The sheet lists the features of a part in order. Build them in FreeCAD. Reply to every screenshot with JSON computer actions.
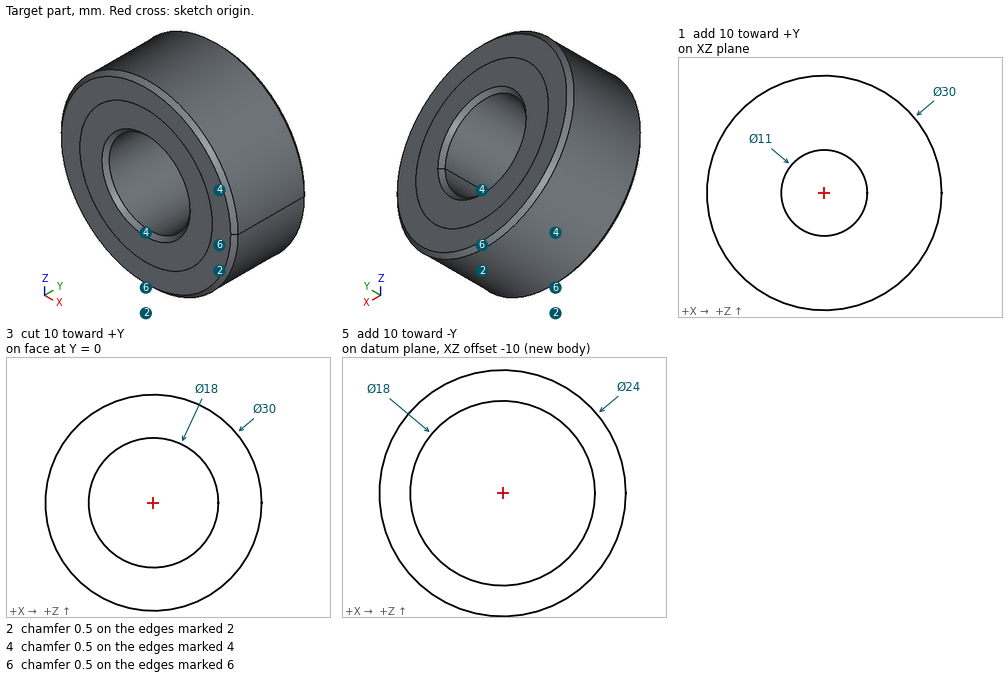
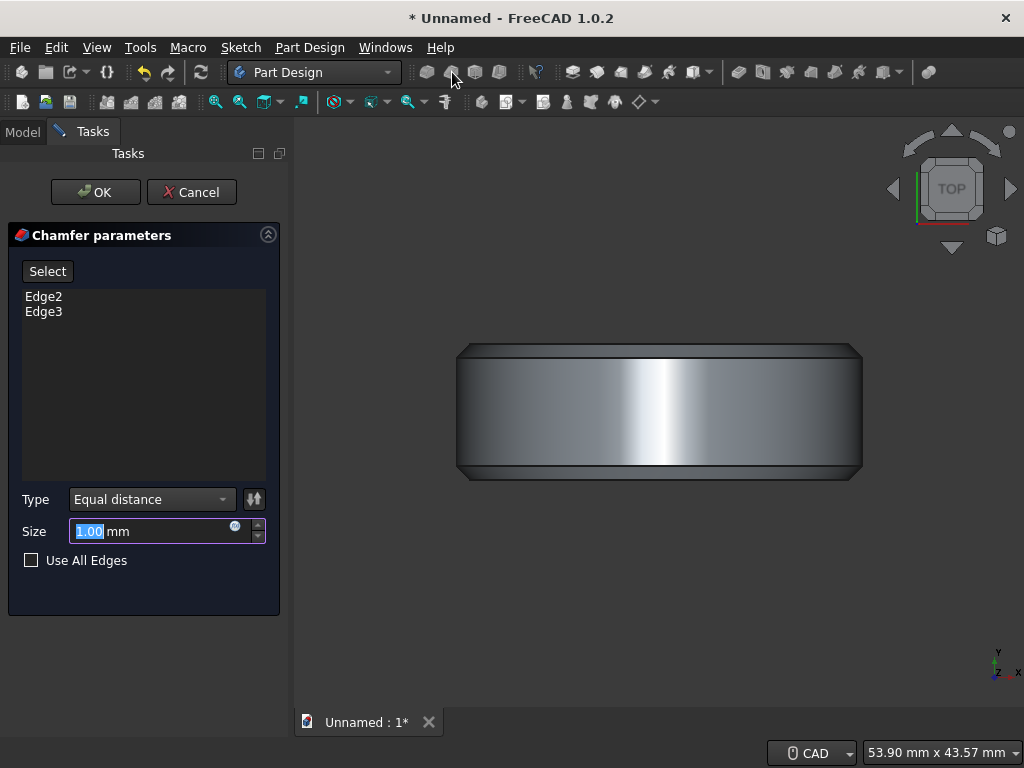
{"action": "type", "text": "0.5"}
{"action": "key", "text": "Tab"}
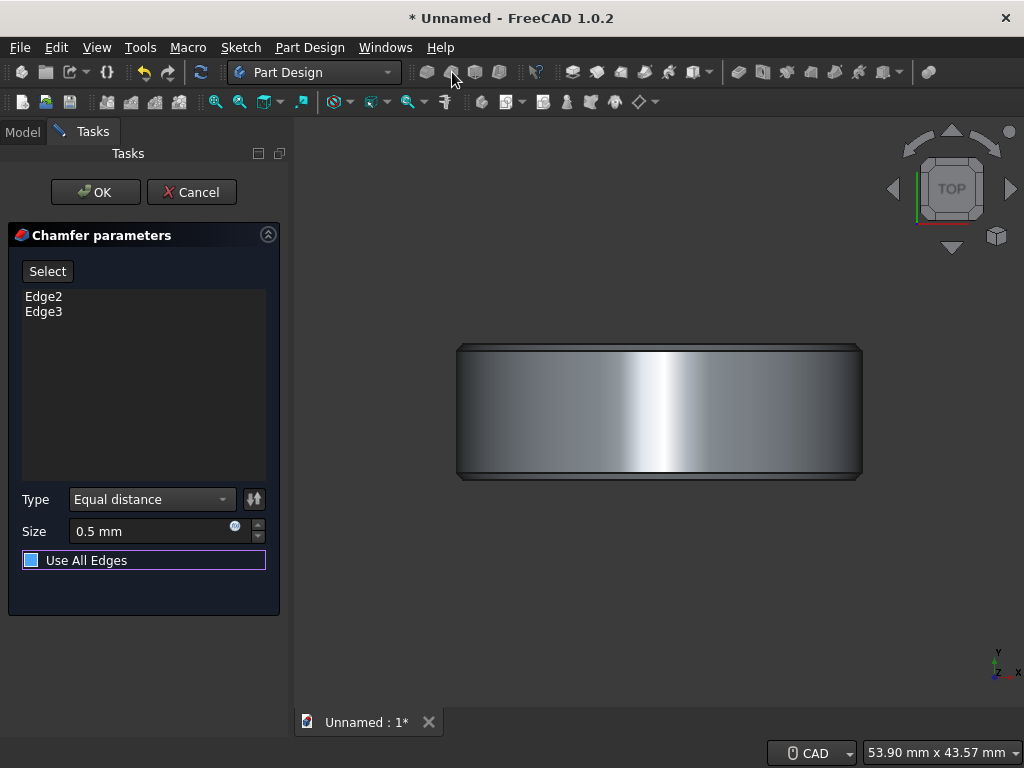
{"action": "left_click", "coordinate": [96, 192]}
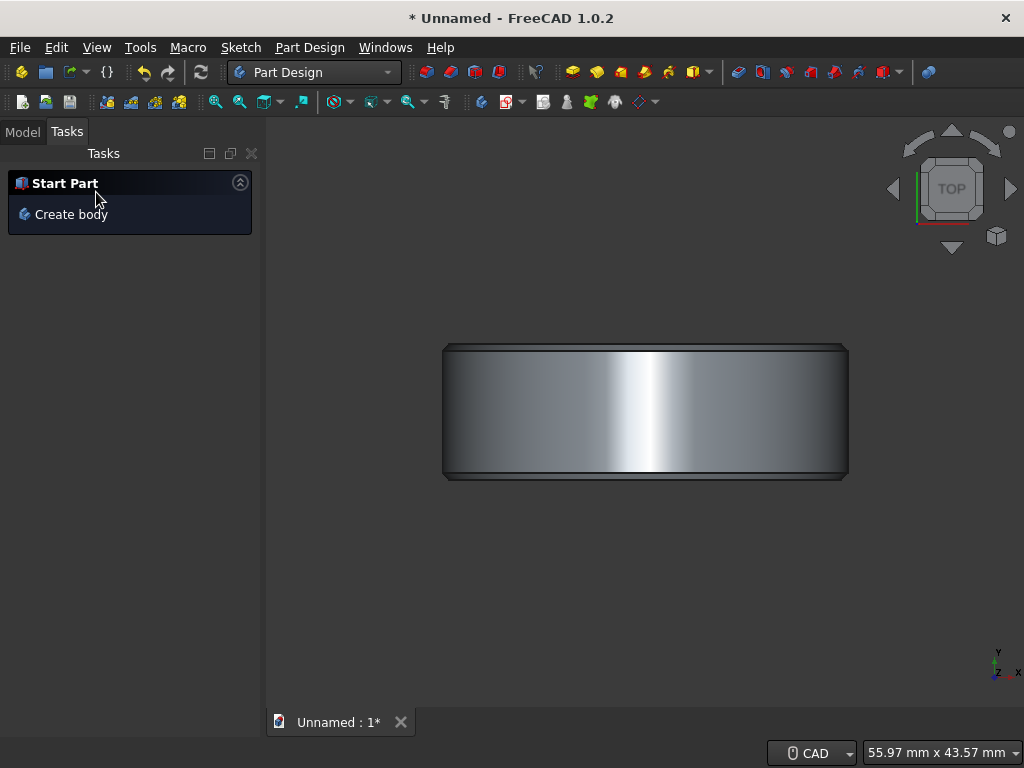
{"action": "key", "text": "0"}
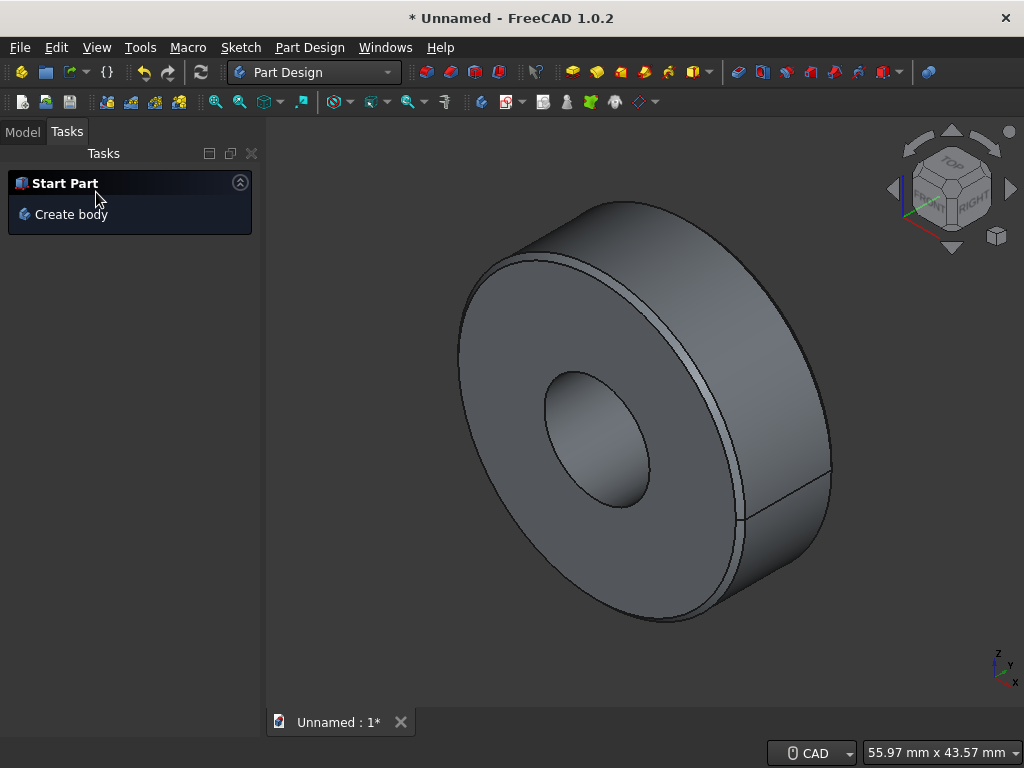
{"action": "left_click", "coordinate": [557, 507]}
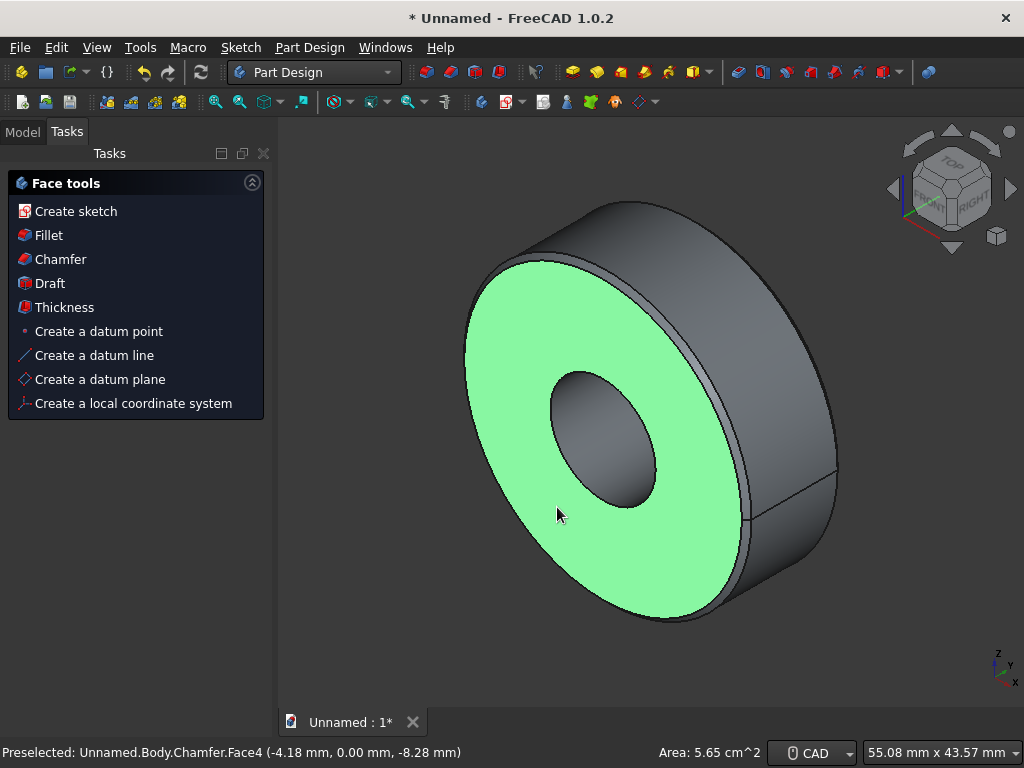
{"action": "left_click", "coordinate": [506, 102]}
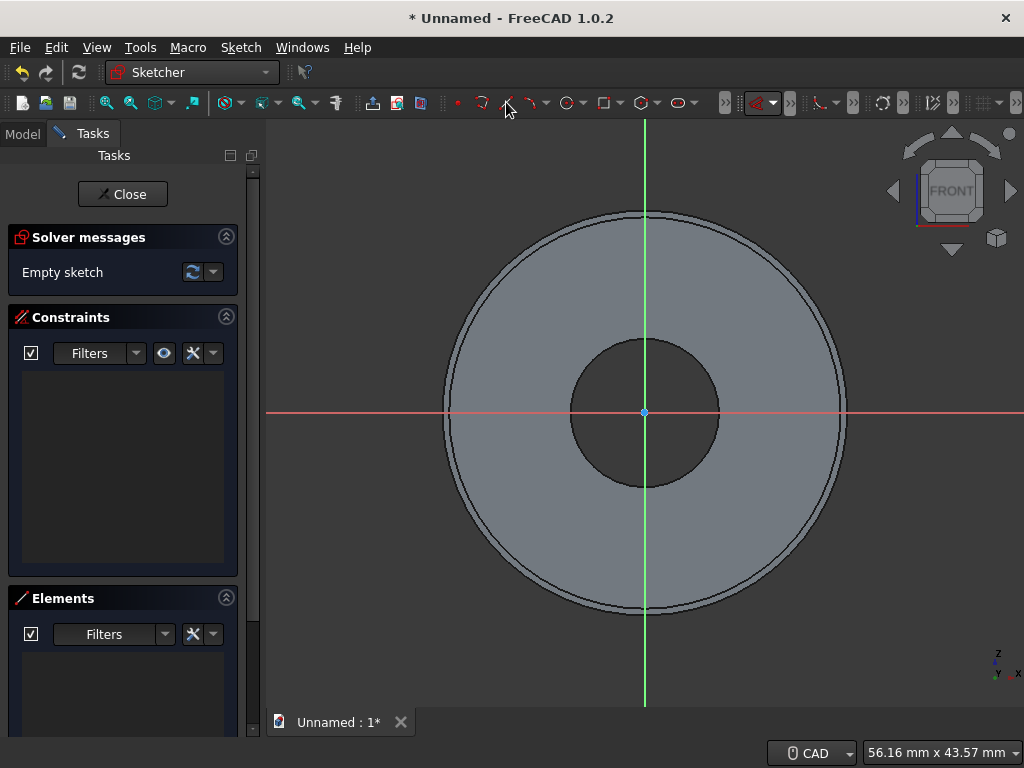
{"action": "scroll", "coordinate": [294, 413], "scroll_direction": "down", "scroll_amount": 1}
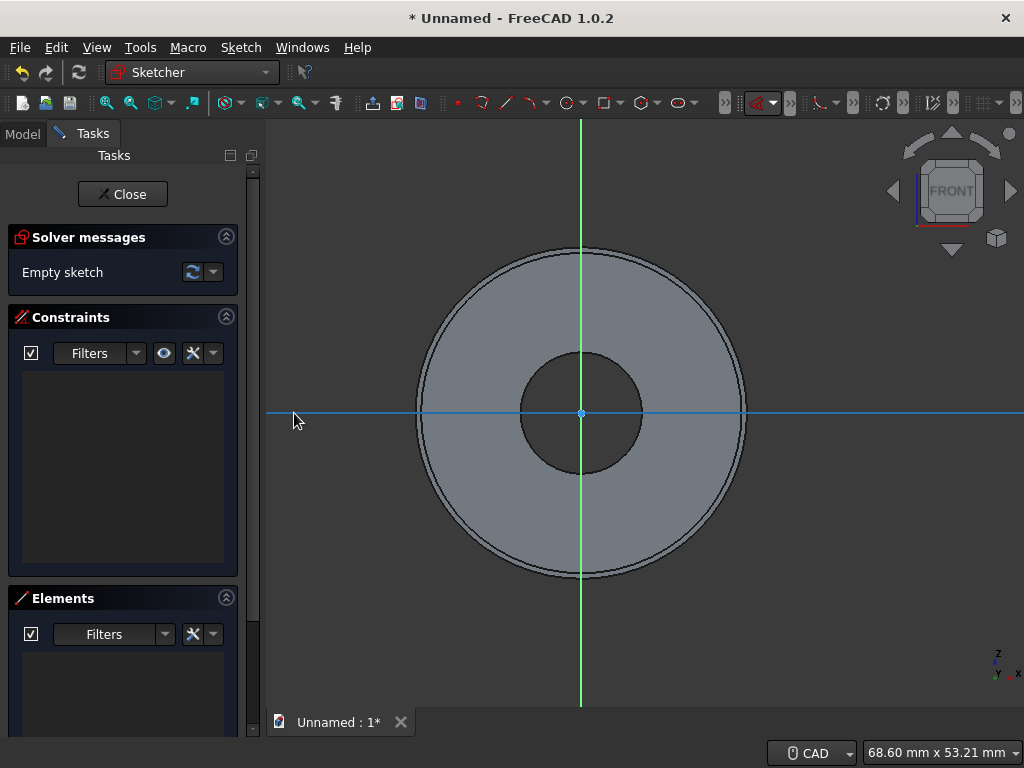
{"action": "left_click", "coordinate": [568, 104]}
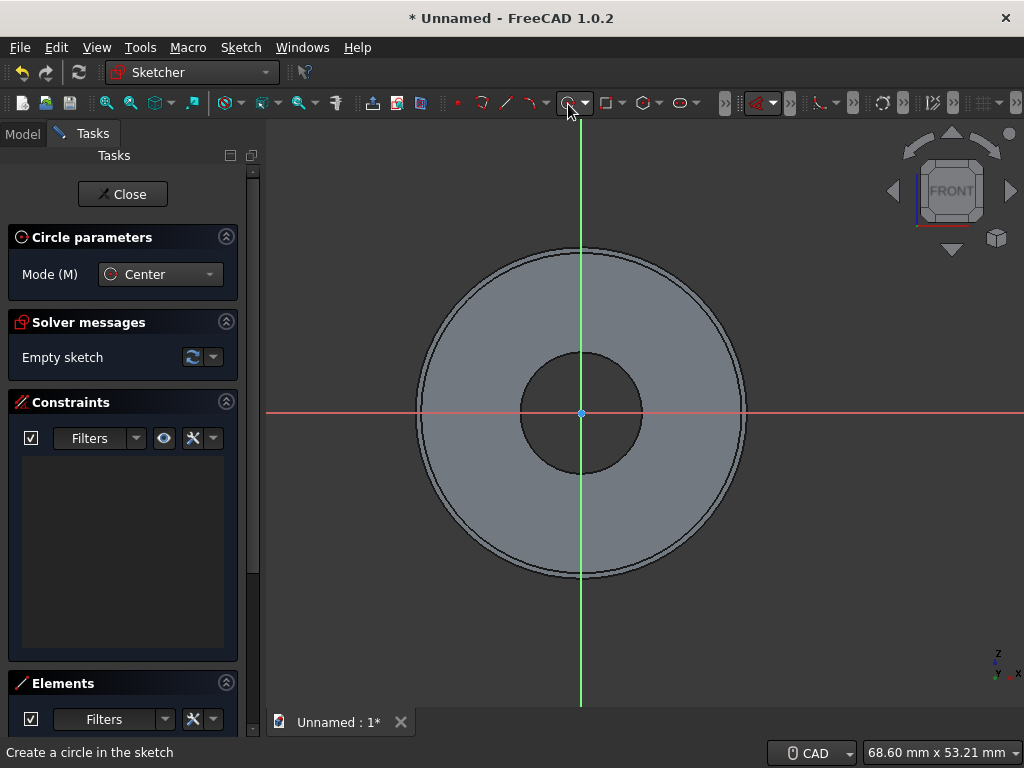
{"action": "left_click", "coordinate": [581, 413]}
{"action": "left_click", "coordinate": [698, 296]}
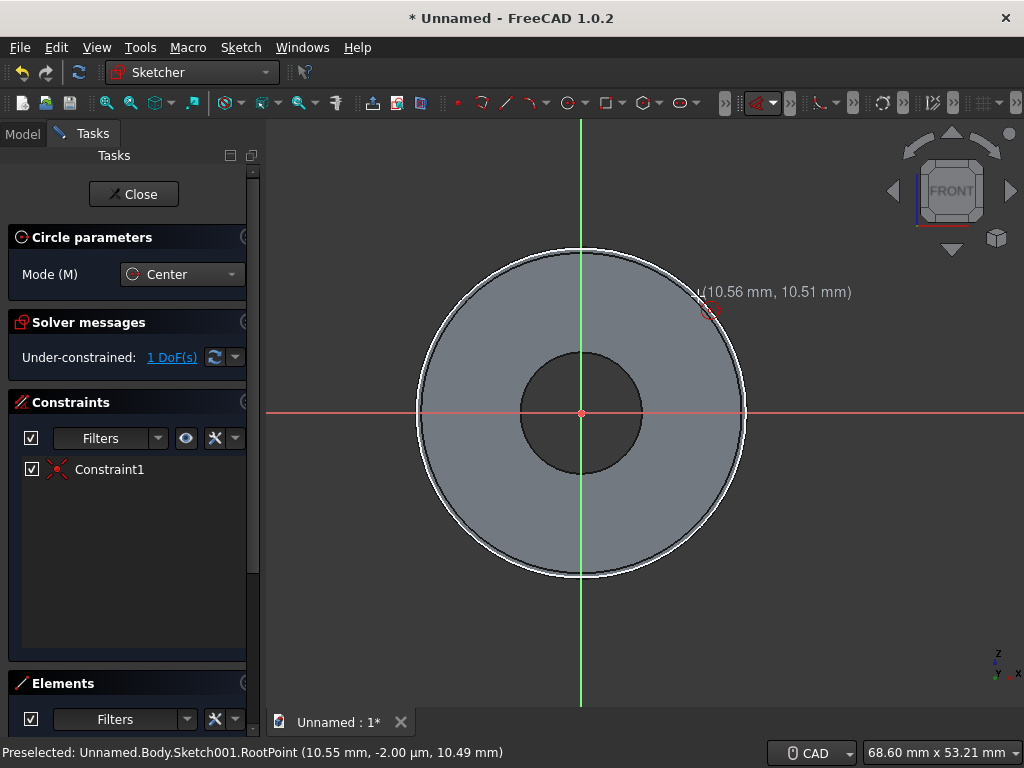
{"action": "left_click", "coordinate": [581, 413]}
{"action": "left_click", "coordinate": [652, 343]}
{"action": "key", "text": "Escape"}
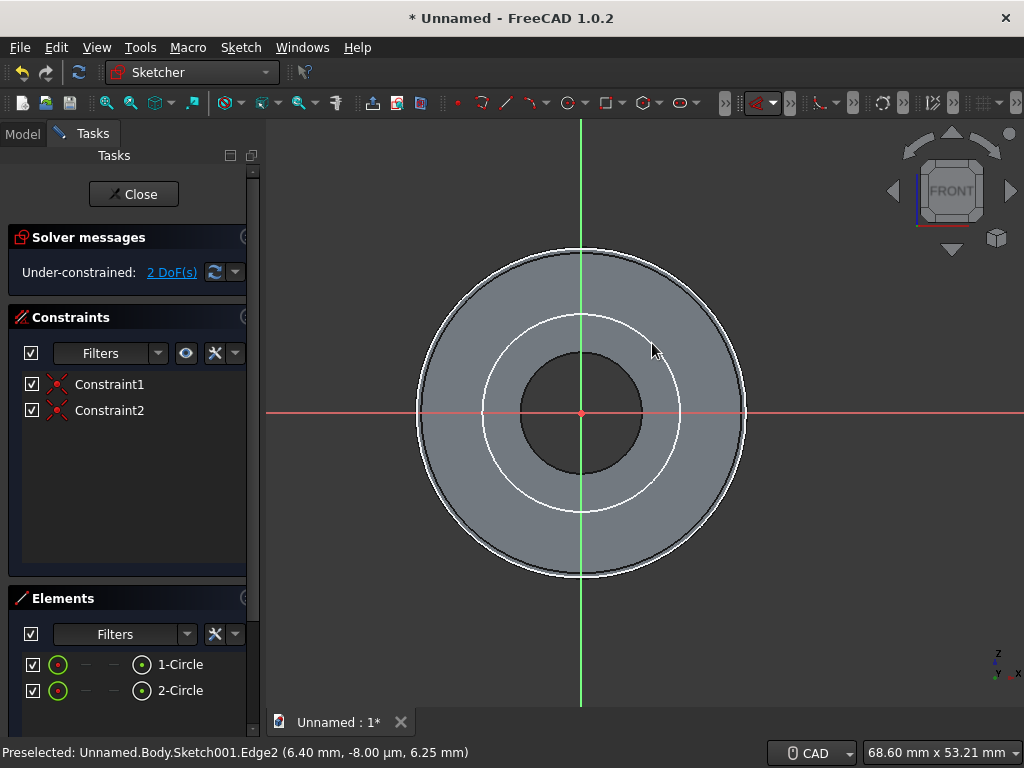
{"action": "left_click", "coordinate": [697, 296]}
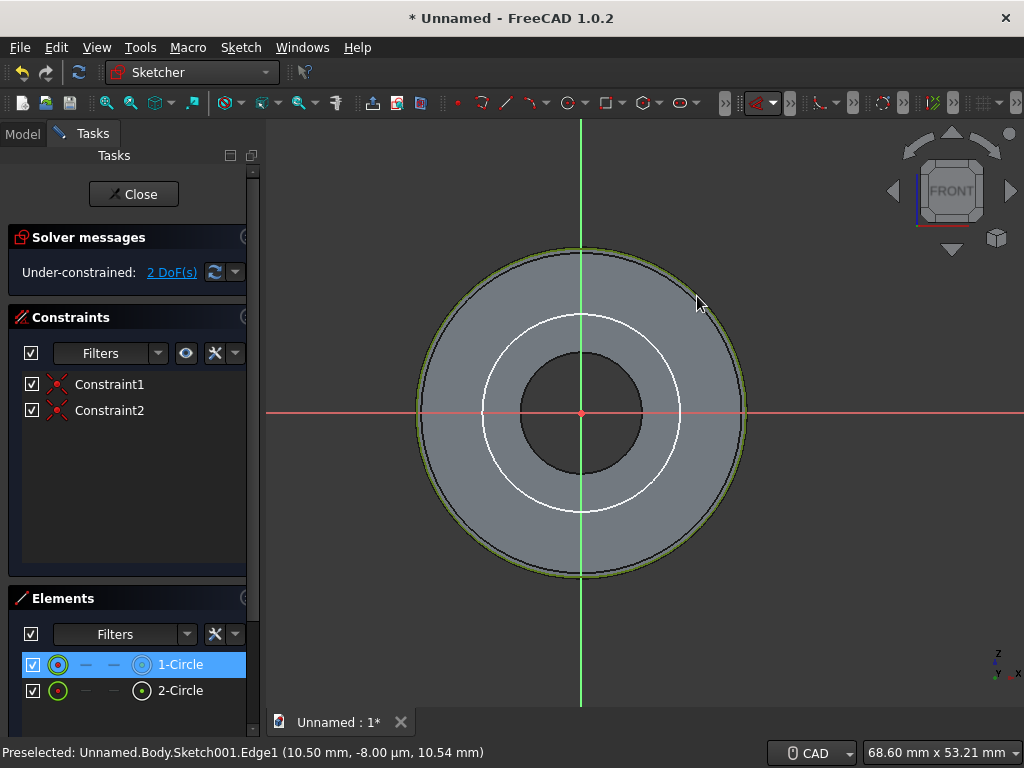
{"action": "left_click", "coordinate": [776, 104]}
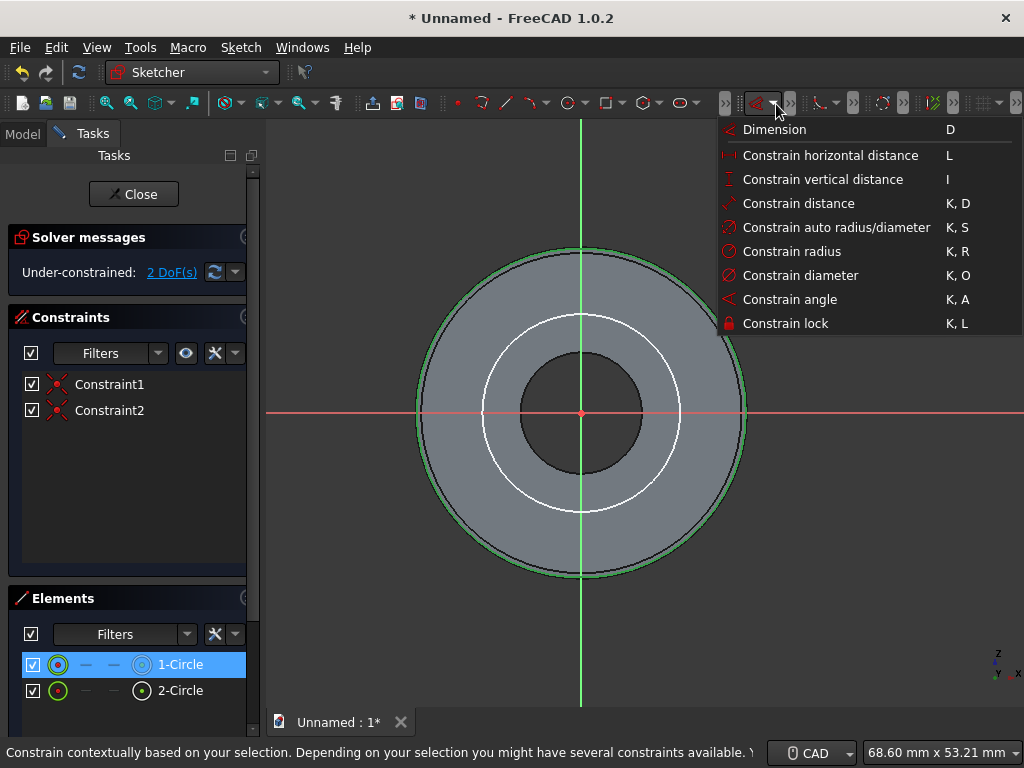
{"action": "left_click", "coordinate": [870, 275]}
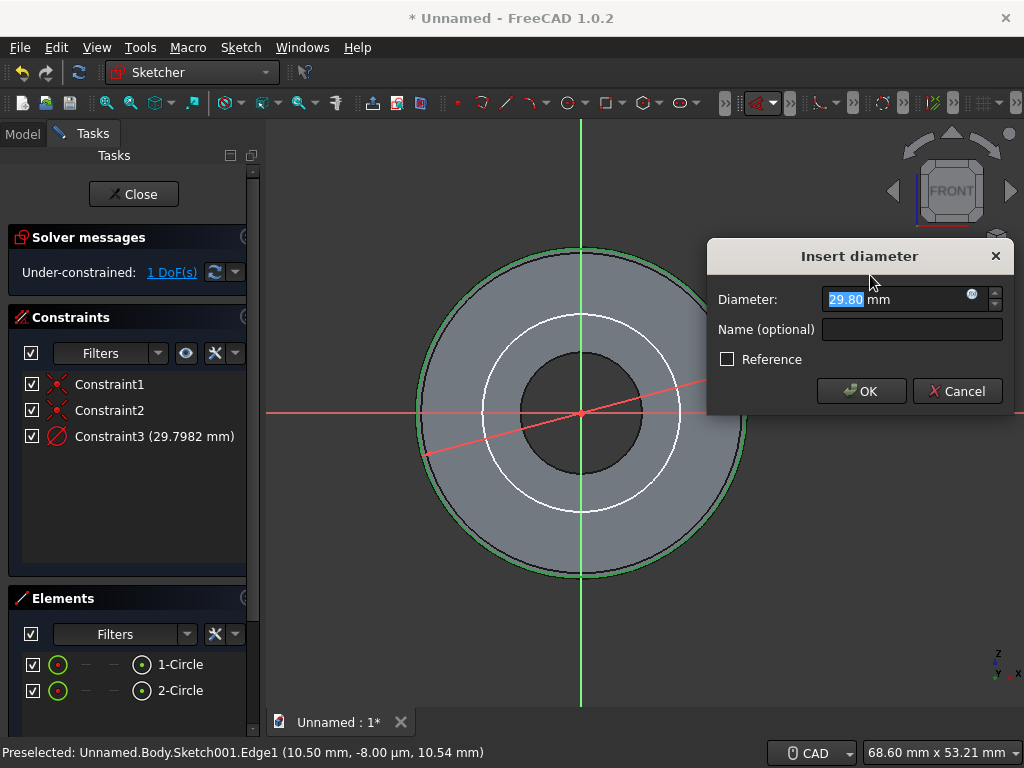
{"action": "type", "text": "30"}
{"action": "key", "text": "Return"}